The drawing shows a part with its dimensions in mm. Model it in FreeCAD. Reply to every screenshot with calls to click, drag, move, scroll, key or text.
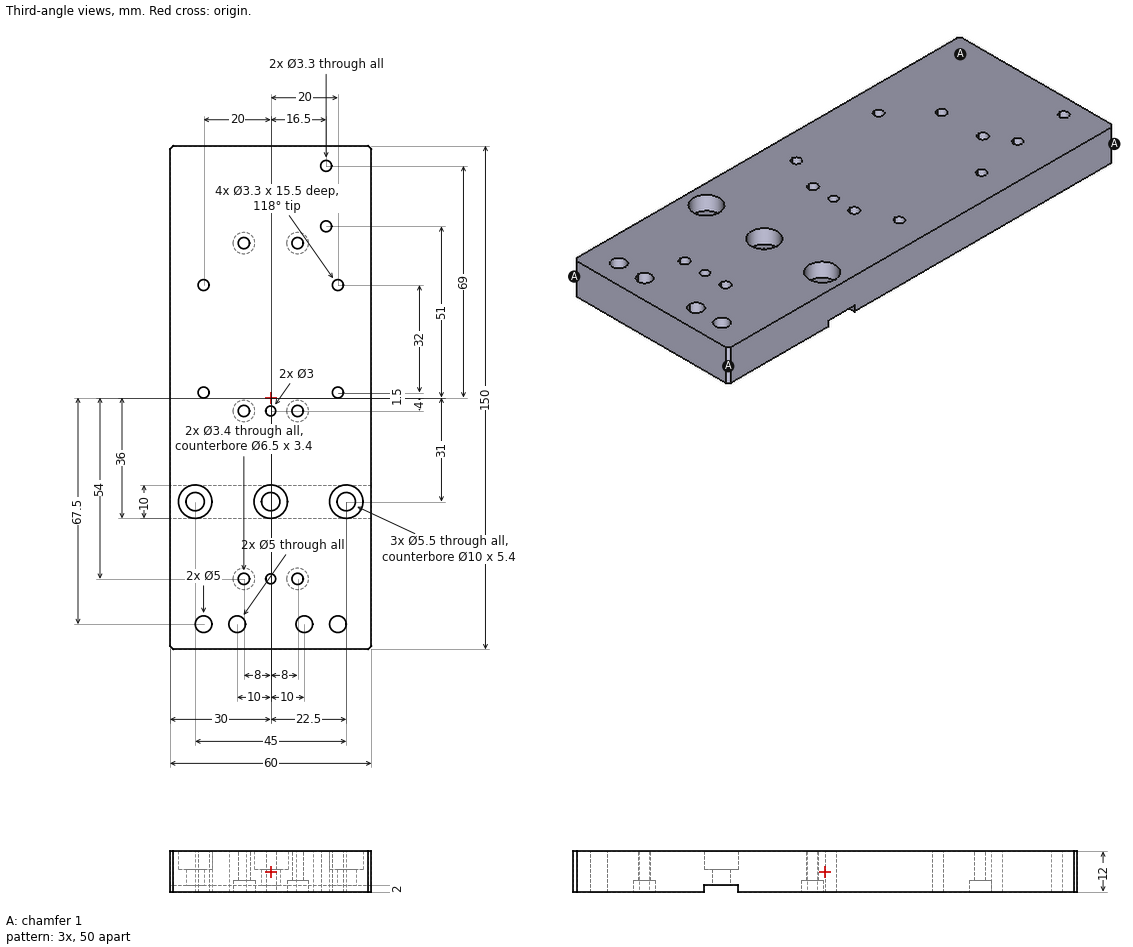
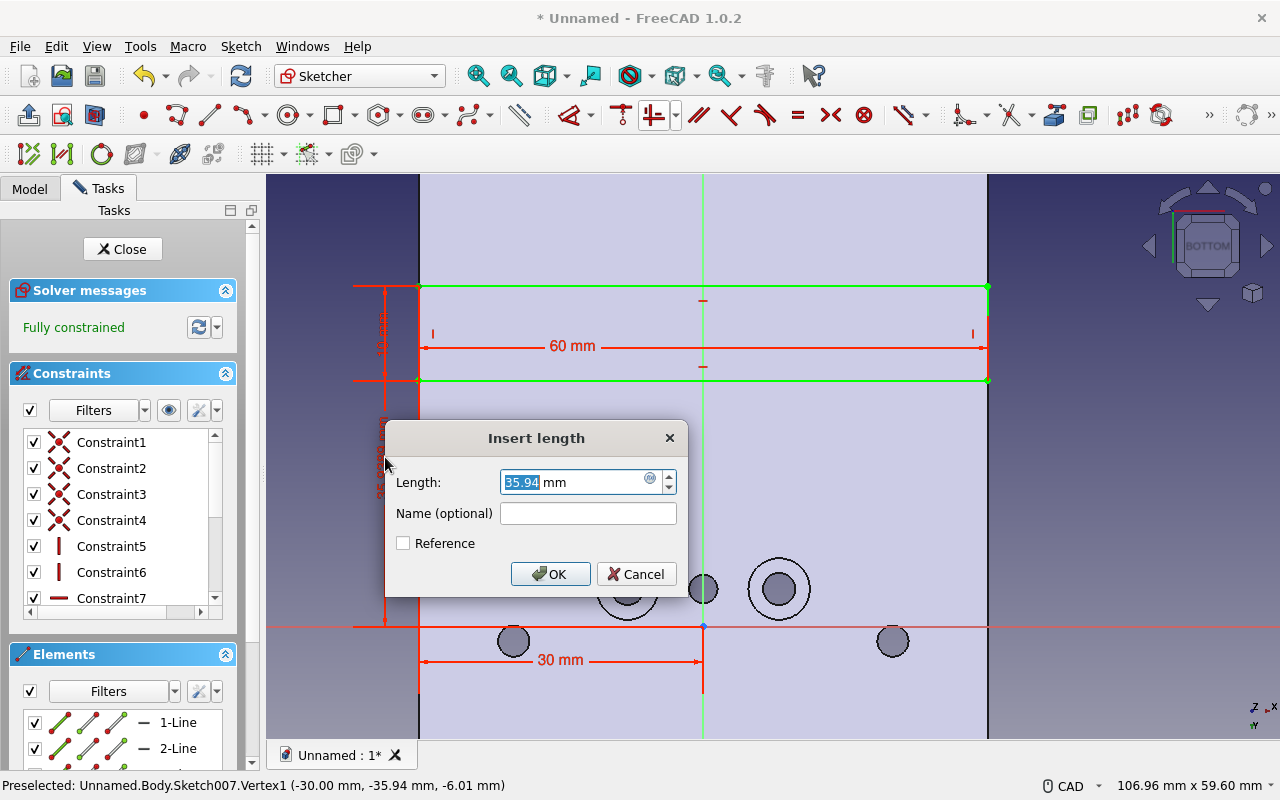
text(36)
key(Return)
key(Escape)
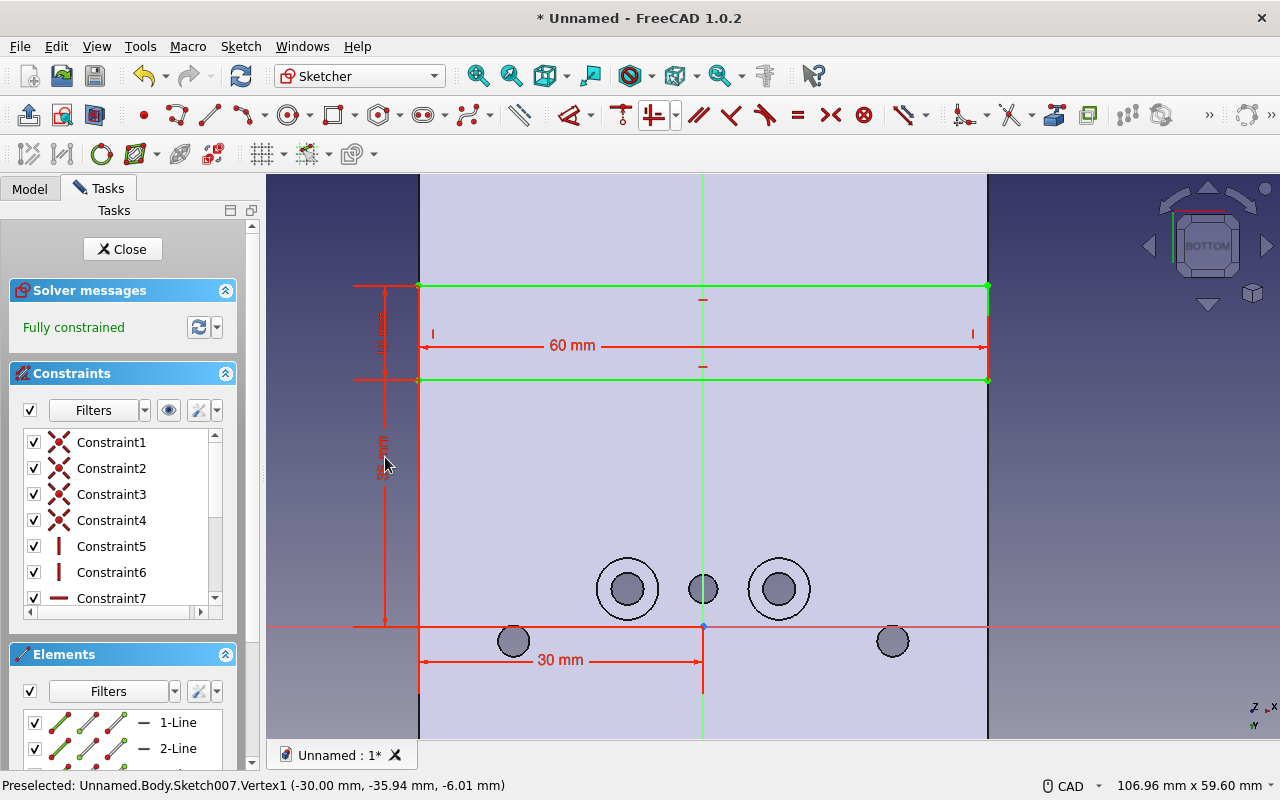
click(123, 249)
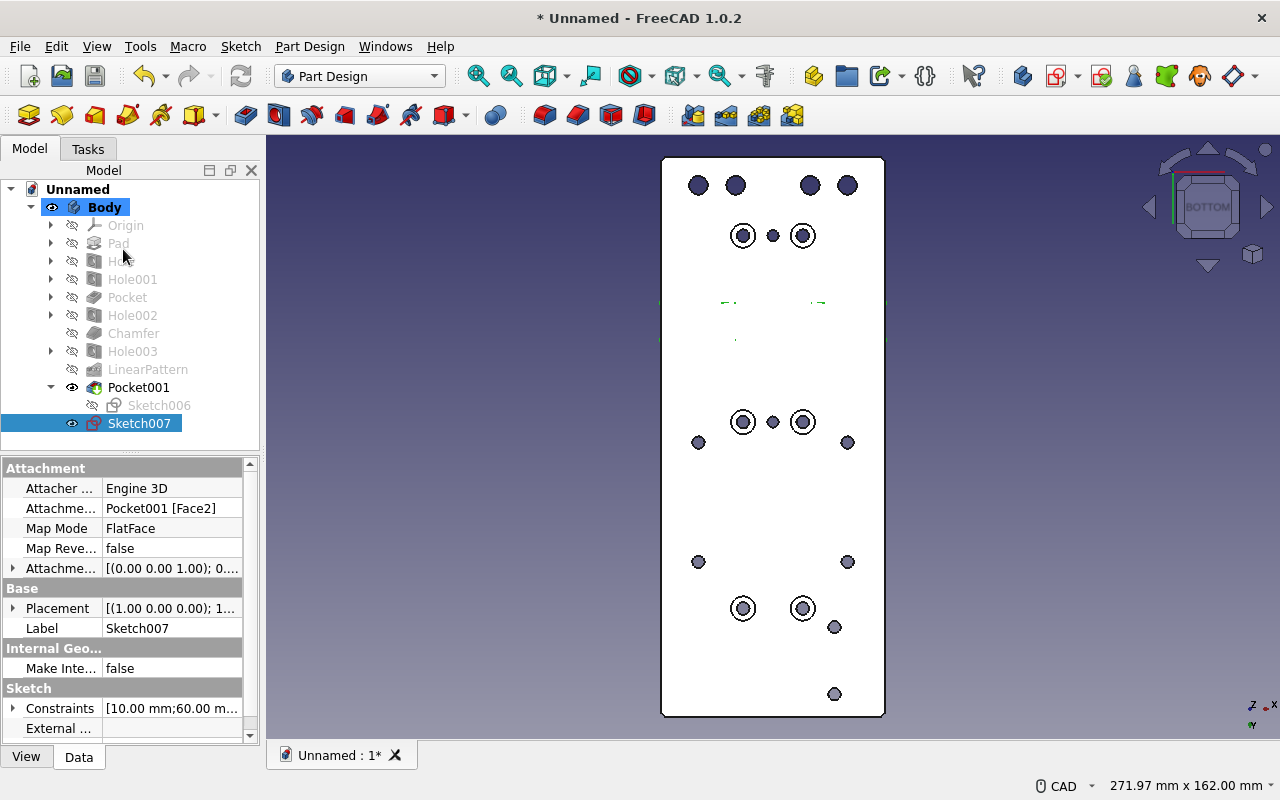
click(246, 116)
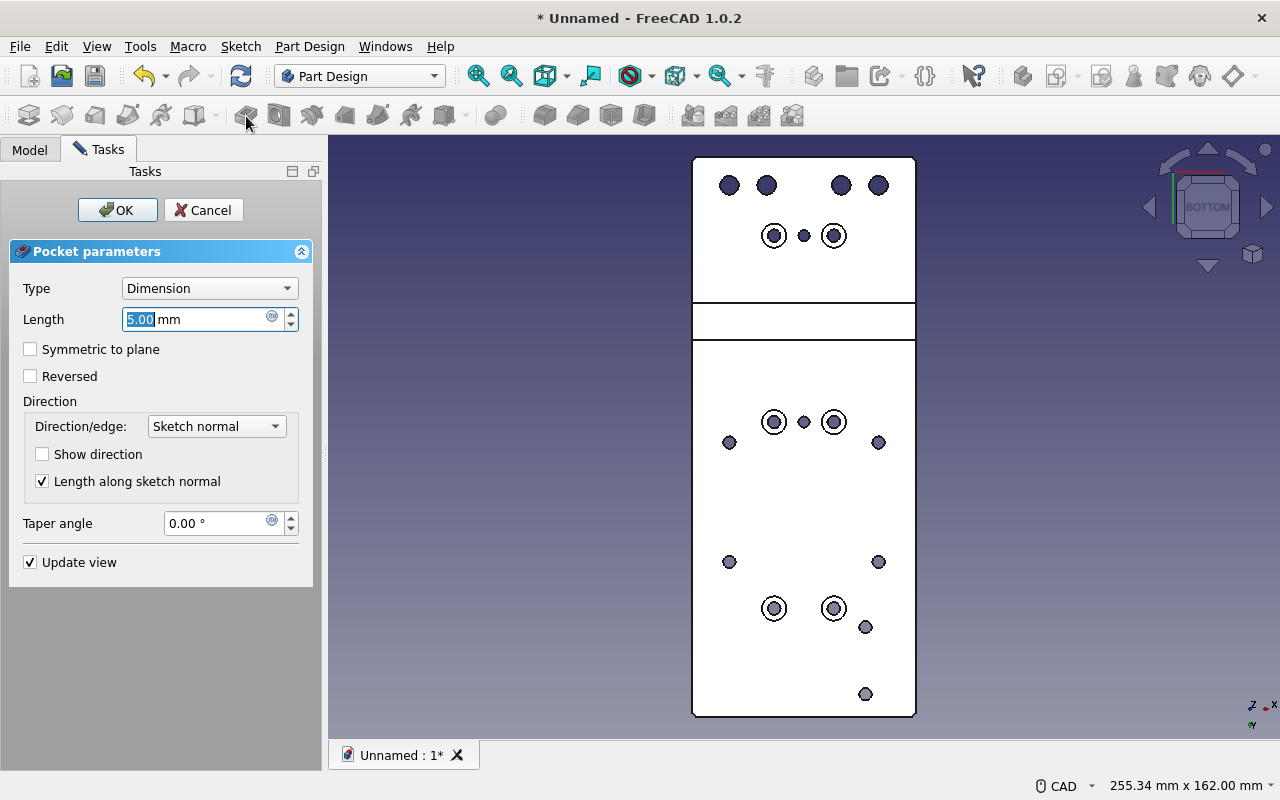
text(2)
key(Tab)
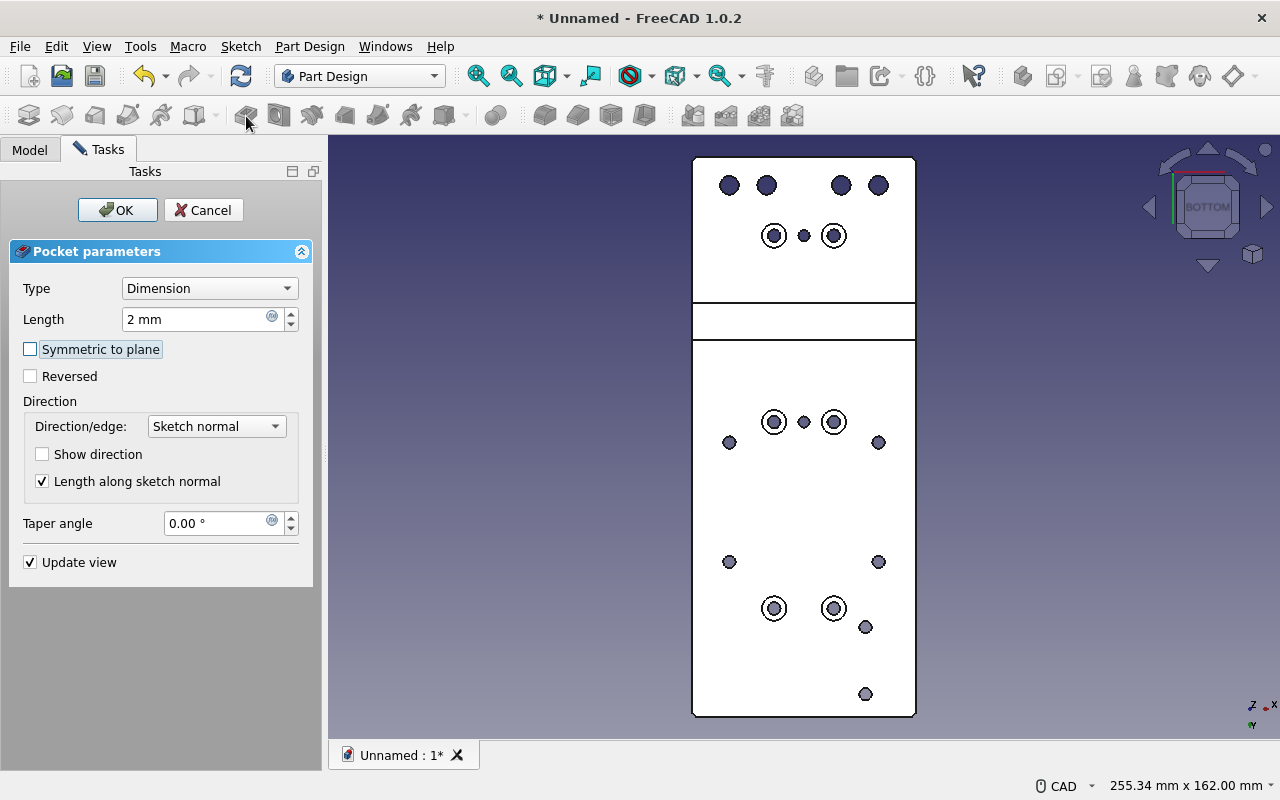
click(118, 210)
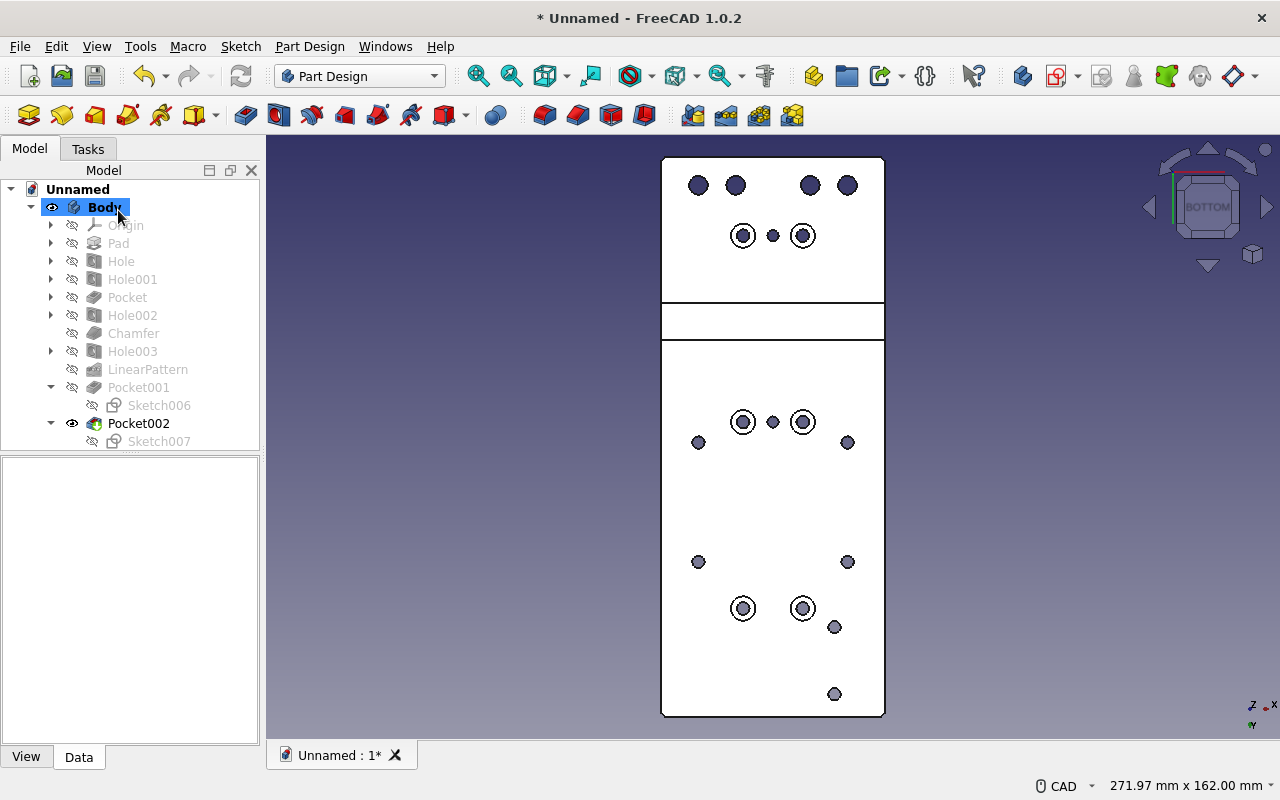
key(0)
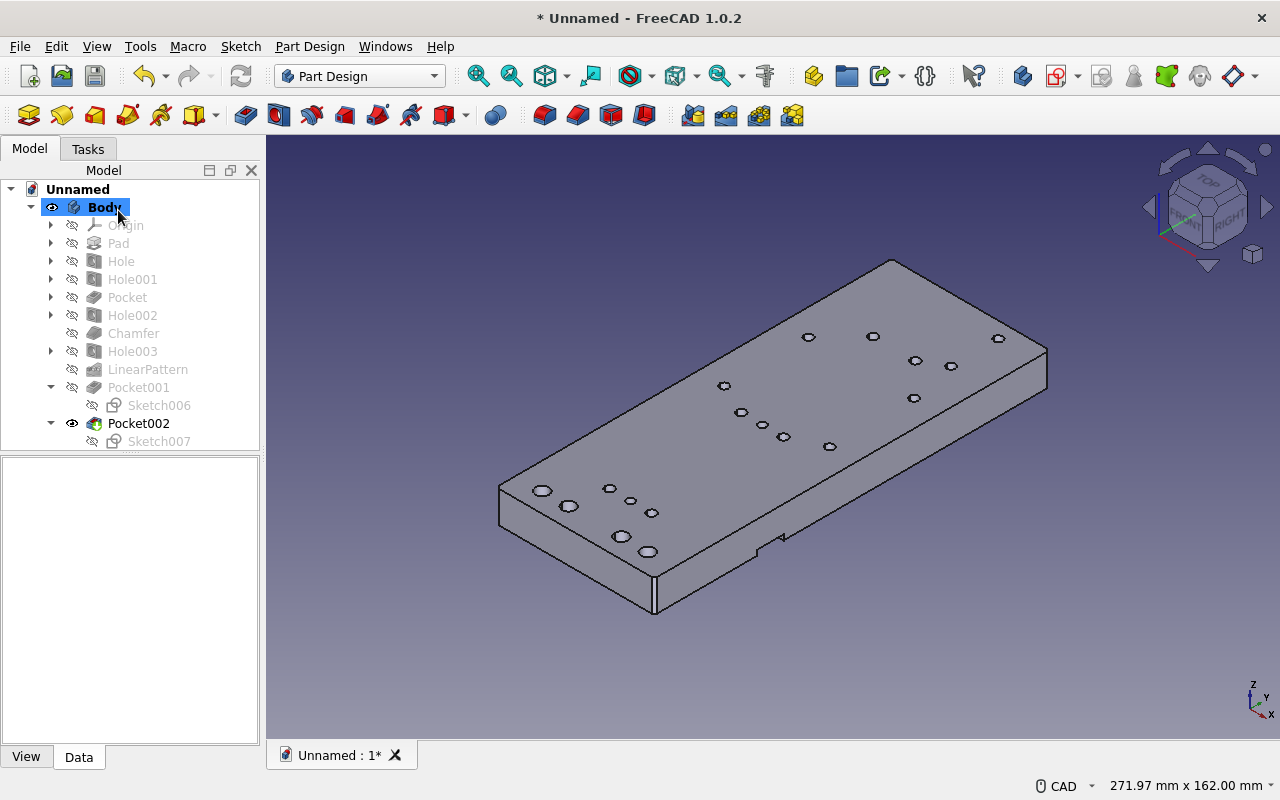
click(829, 385)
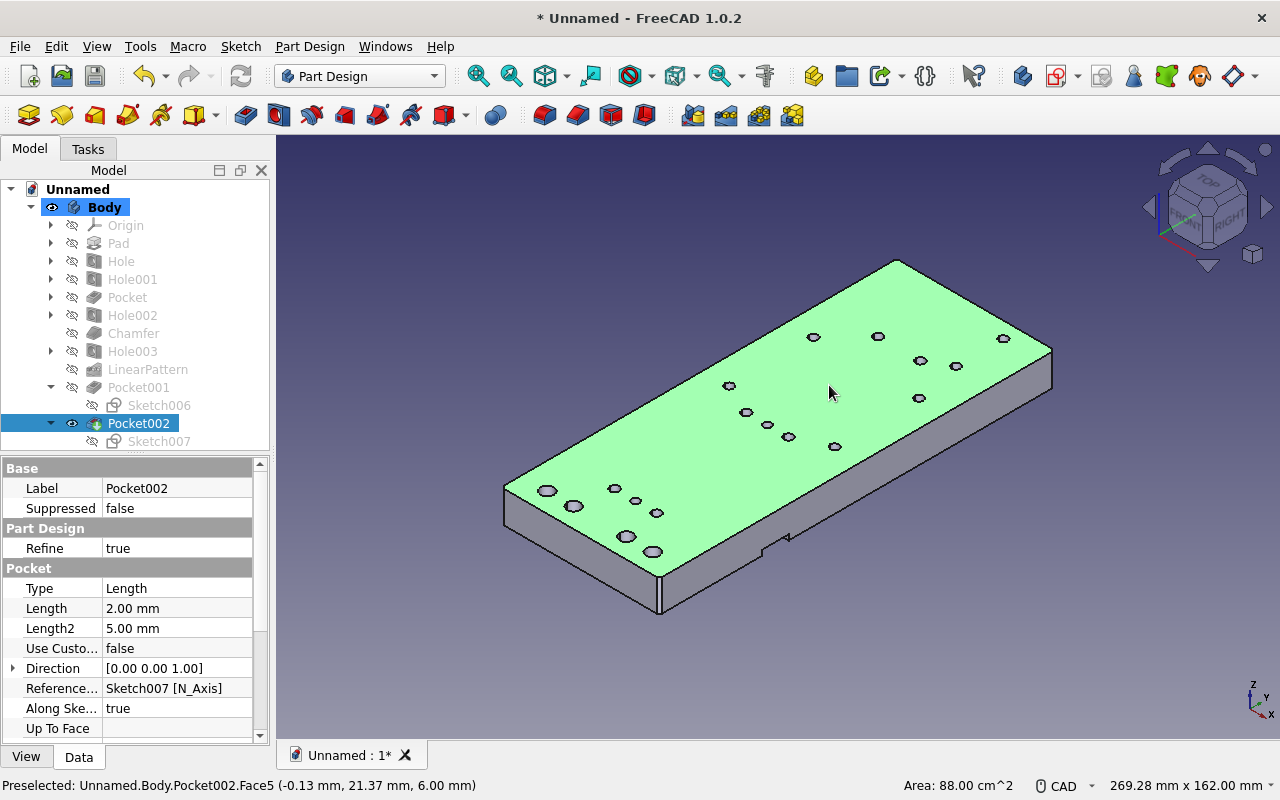
click(1056, 76)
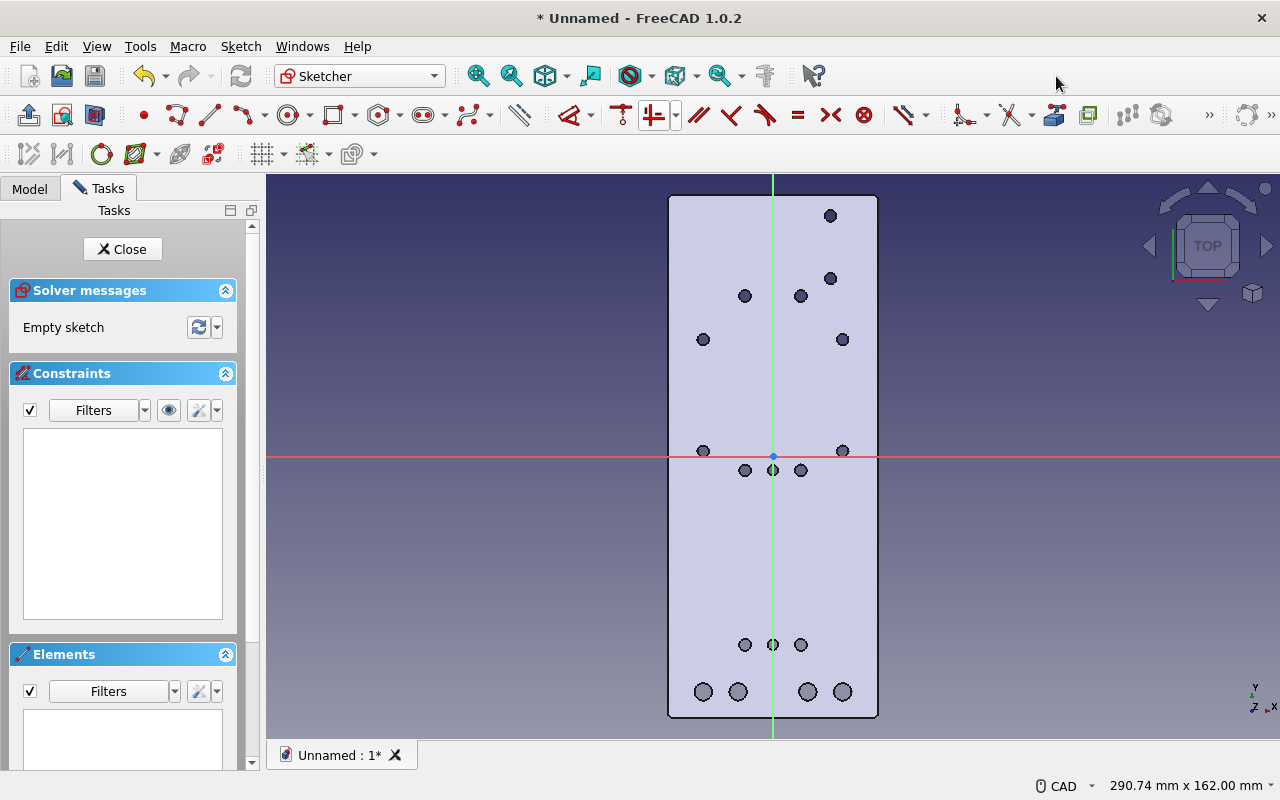
scroll(803, 541, up, 6)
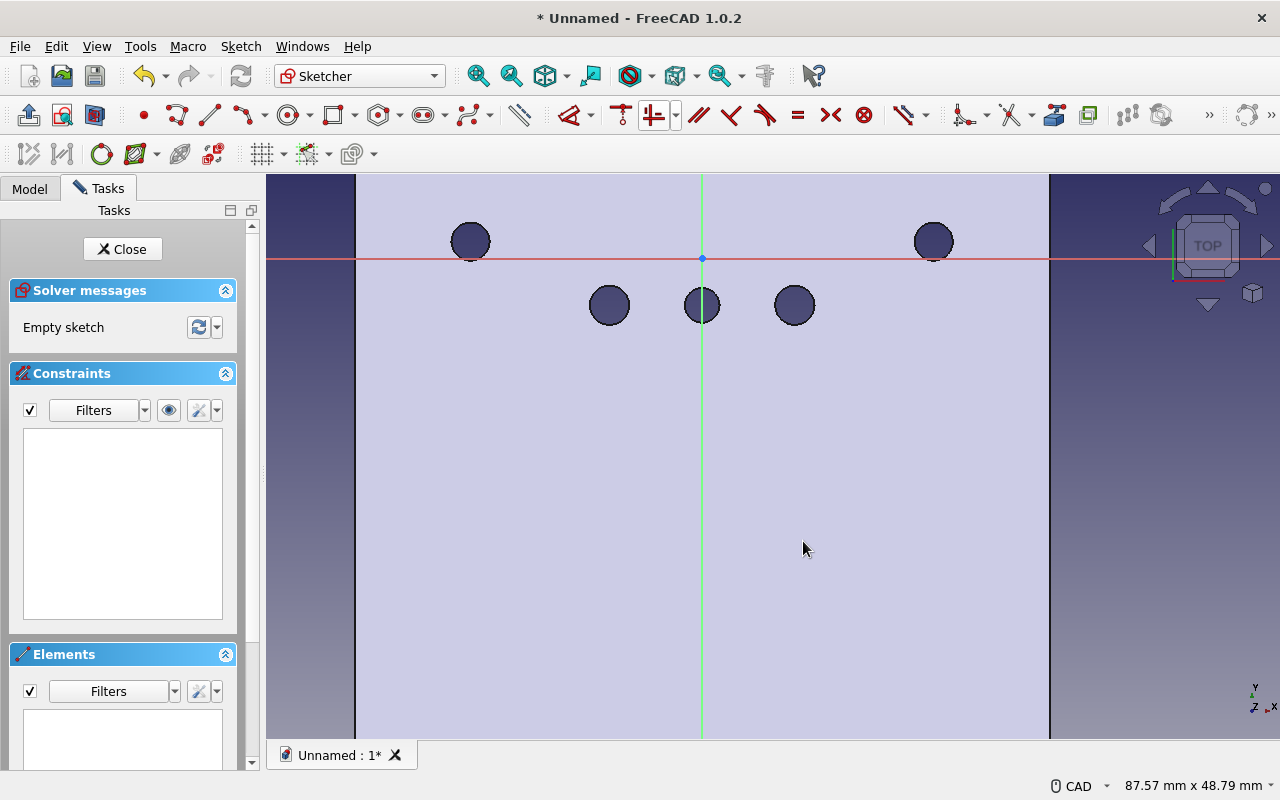
click(288, 116)